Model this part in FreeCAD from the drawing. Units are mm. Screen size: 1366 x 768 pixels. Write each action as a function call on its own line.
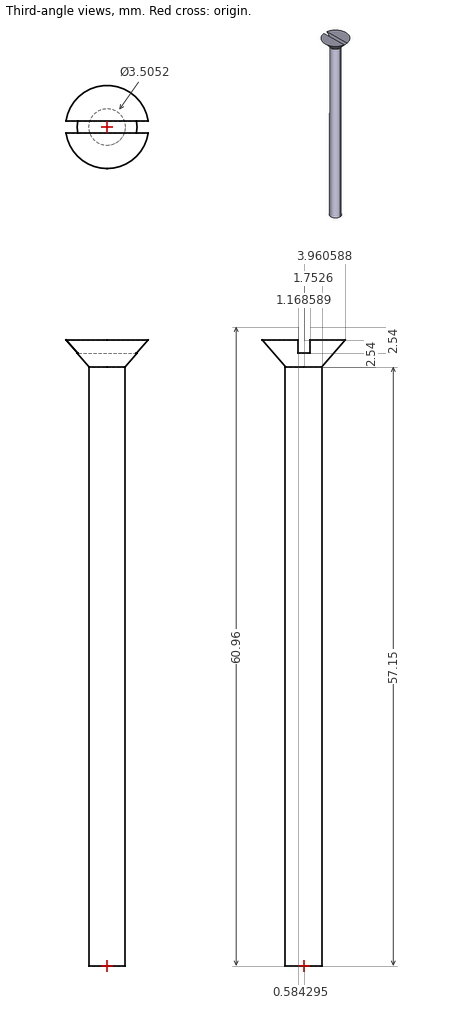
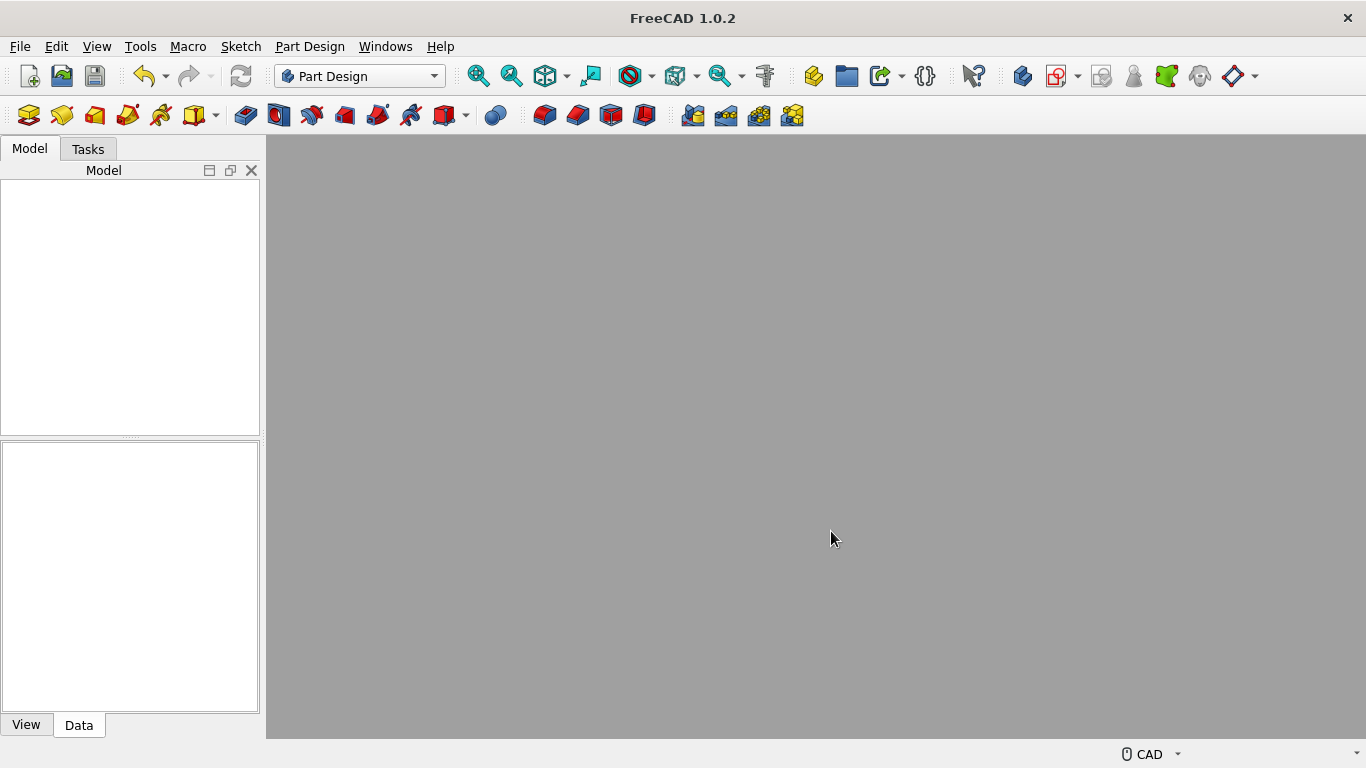
click(29, 76)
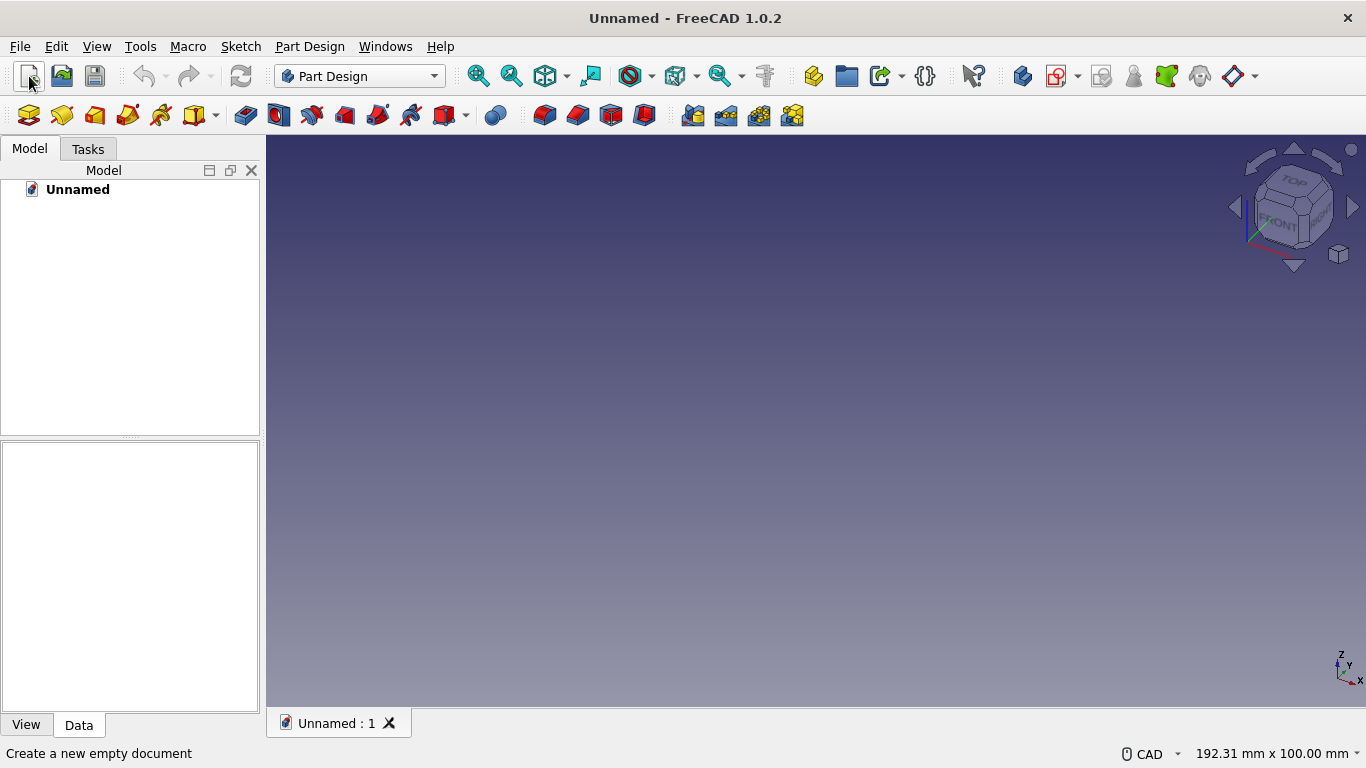
click(1056, 76)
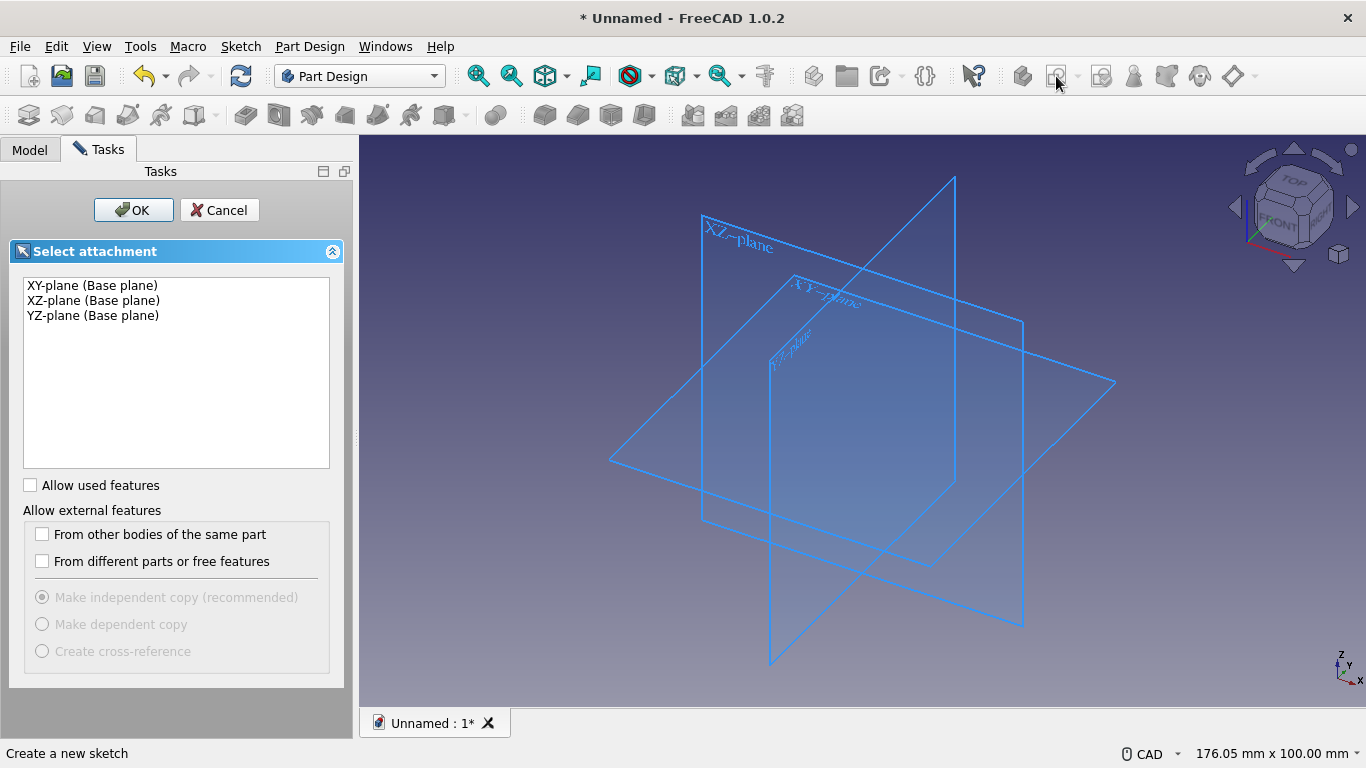
click(84, 286)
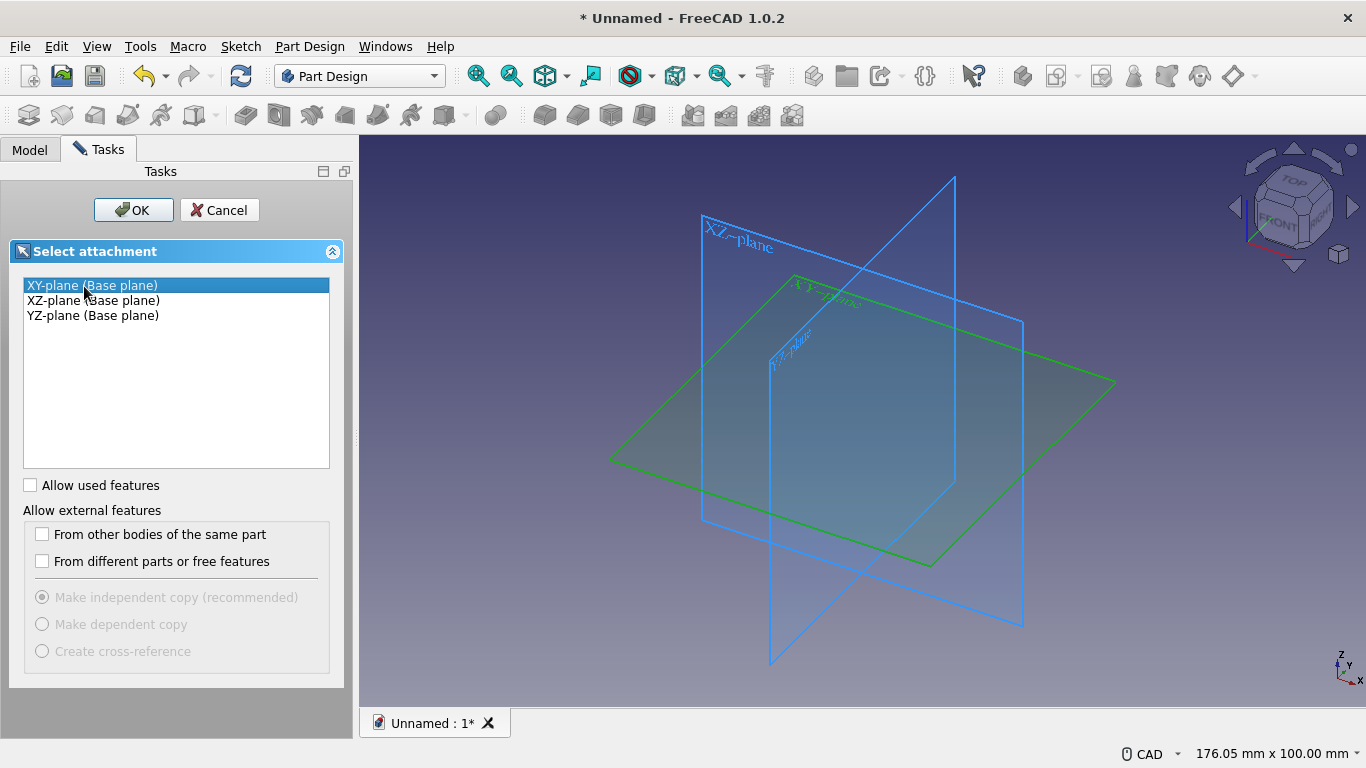
click(134, 210)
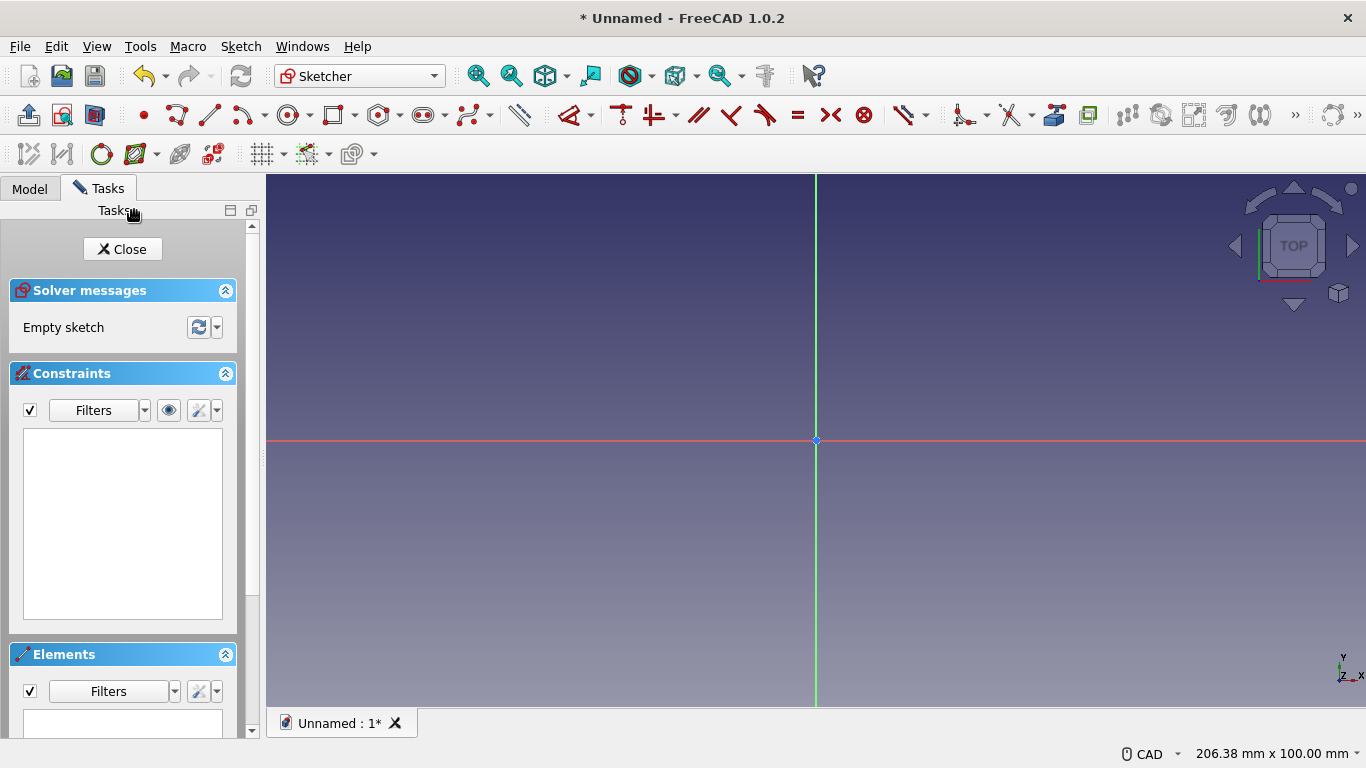
scroll(820, 440, up, 14)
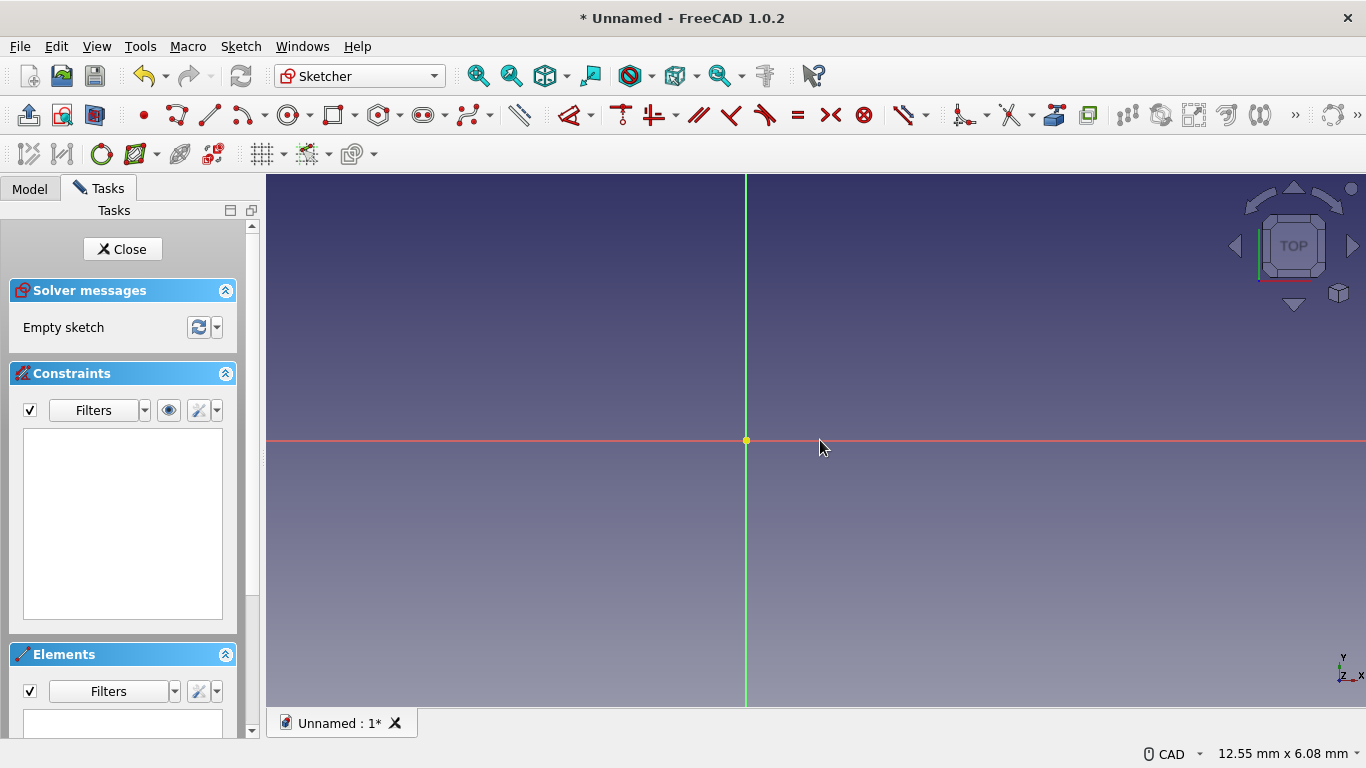
click(288, 116)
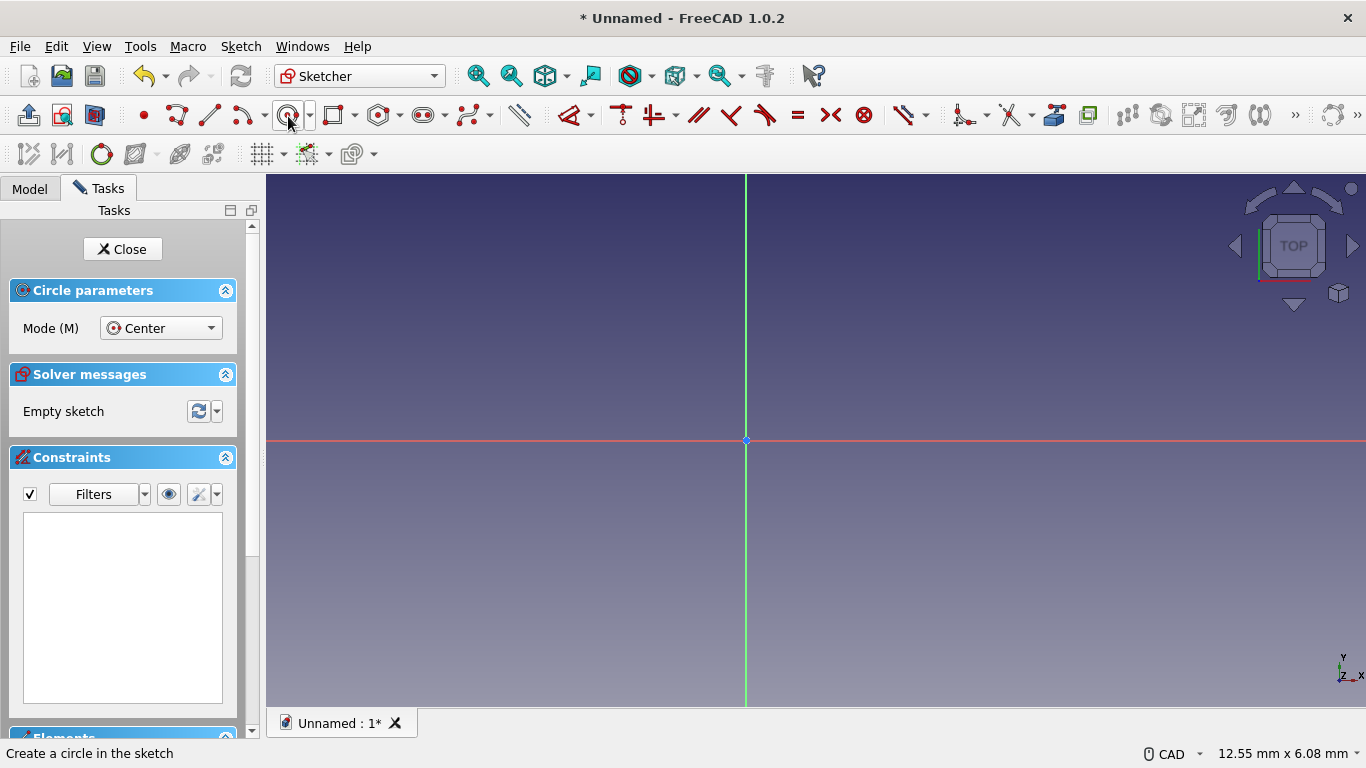
click(746, 440)
move(855, 332)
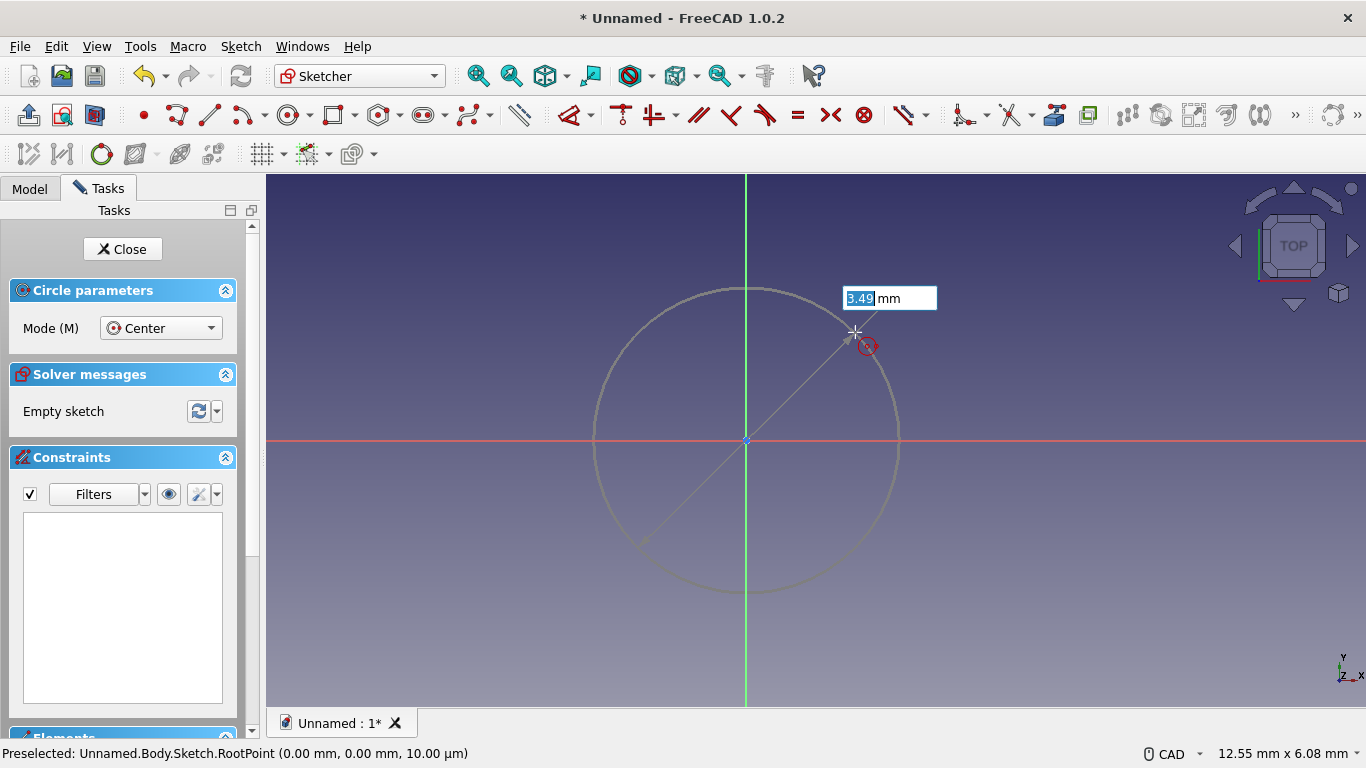
text(3.5052)
key(Return)
key(Escape)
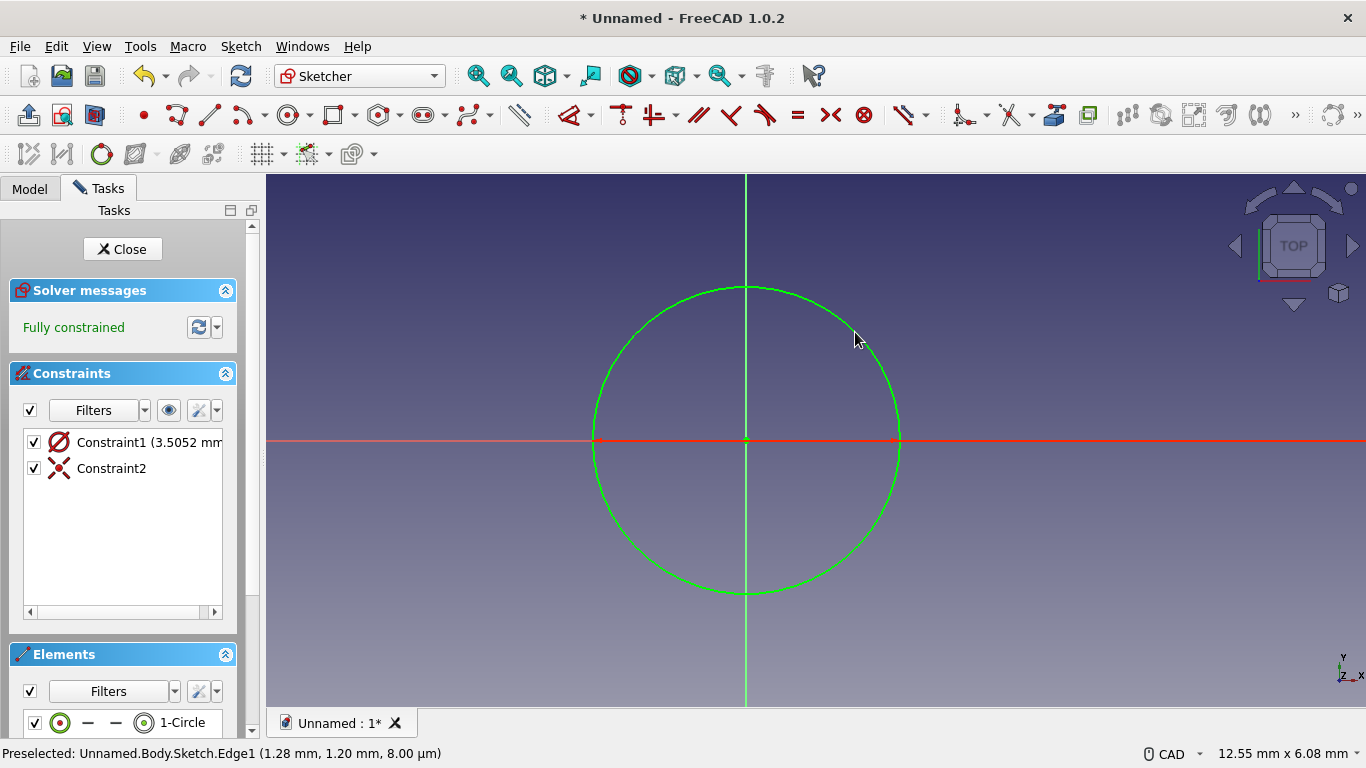
click(123, 249)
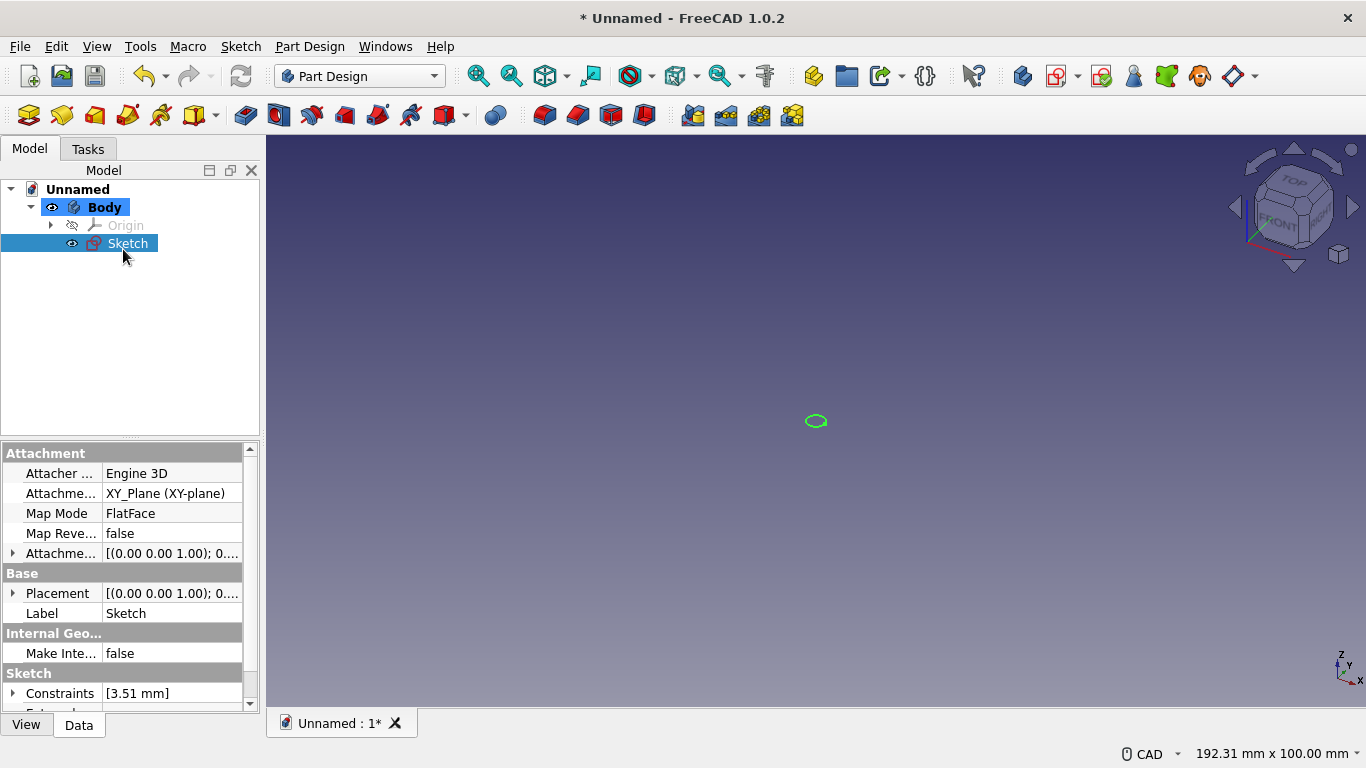
click(29, 116)